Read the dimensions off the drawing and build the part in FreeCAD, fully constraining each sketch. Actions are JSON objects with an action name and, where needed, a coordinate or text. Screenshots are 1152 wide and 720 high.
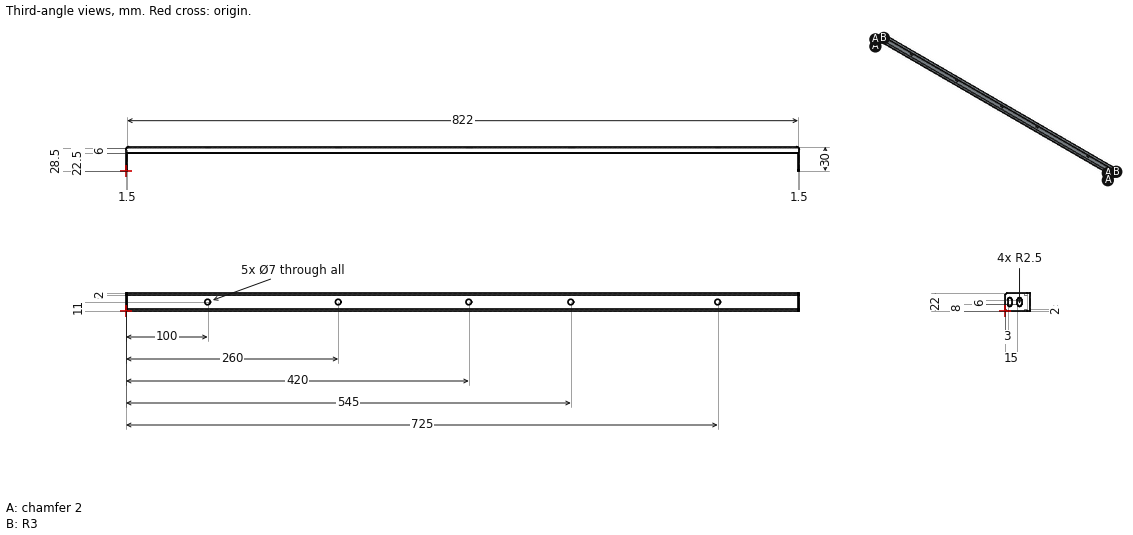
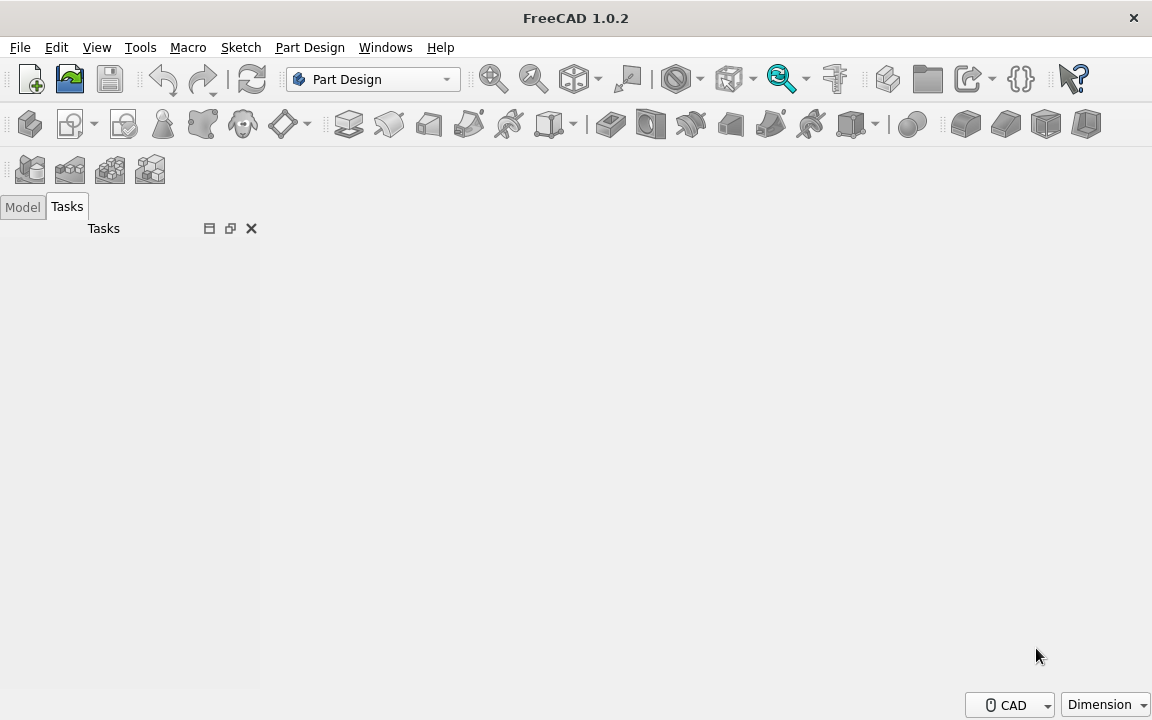
{"action": "left_click", "coordinate": [30, 80]}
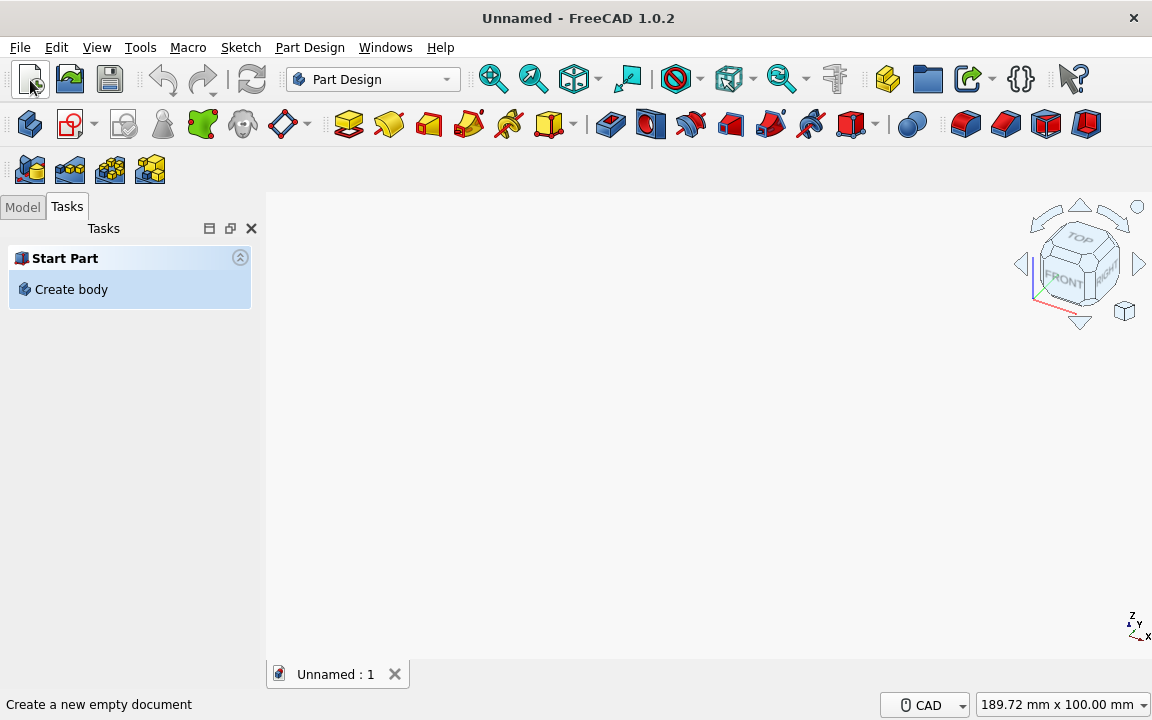
{"action": "left_click", "coordinate": [70, 124]}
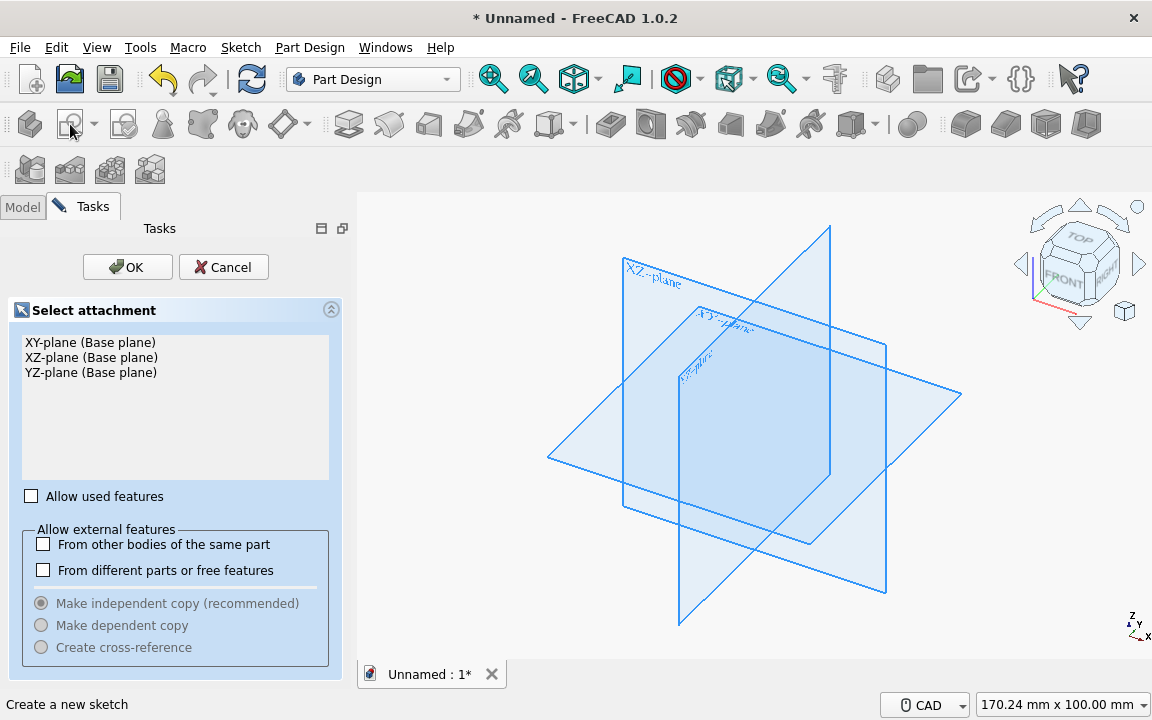
{"action": "left_click", "coordinate": [82, 342]}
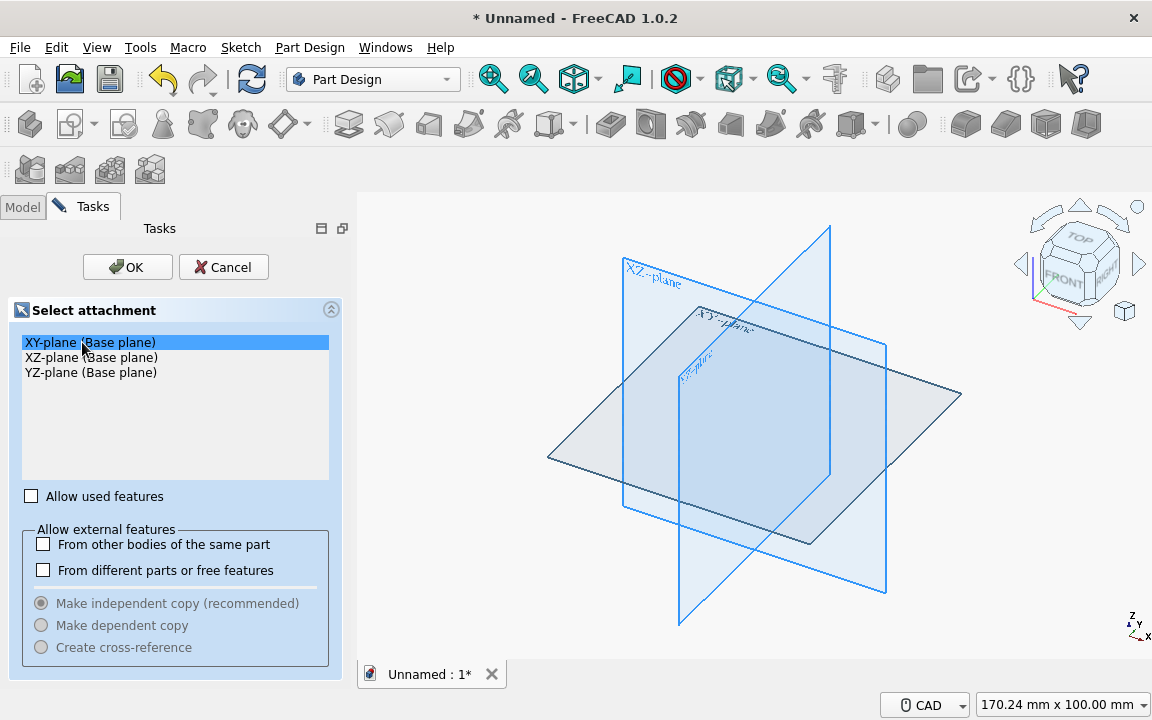
{"action": "left_click", "coordinate": [128, 267]}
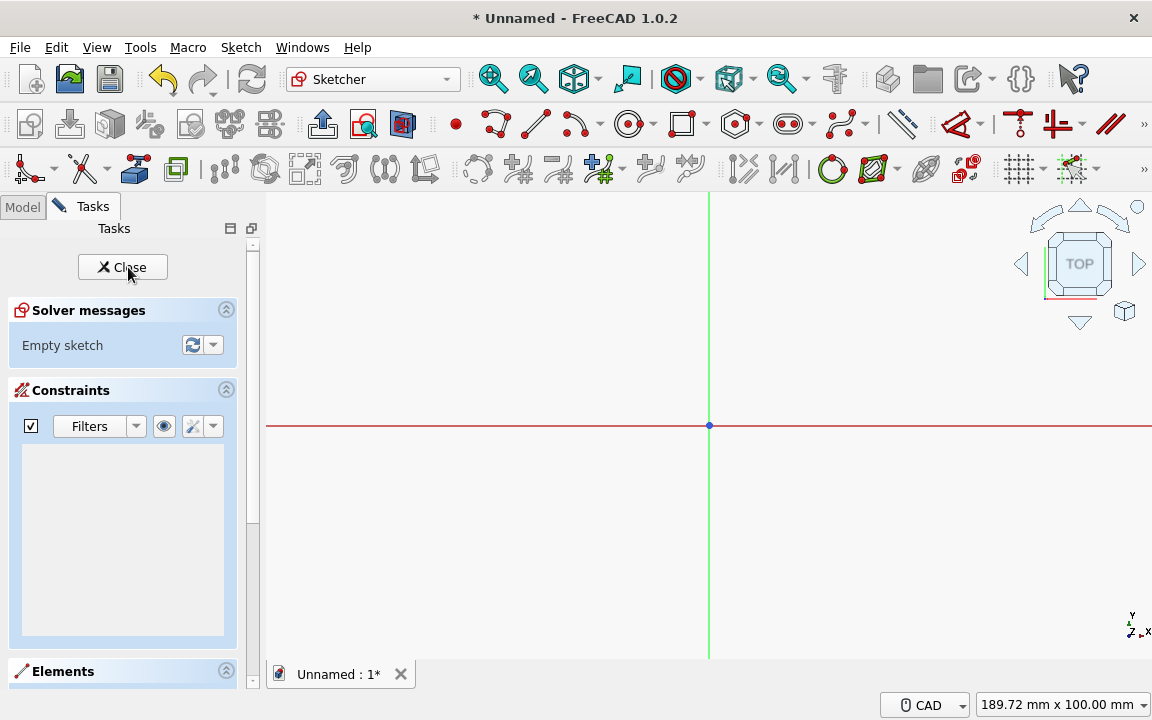
{"action": "scroll", "coordinate": [328, 436], "scroll_direction": "down", "scroll_amount": 10}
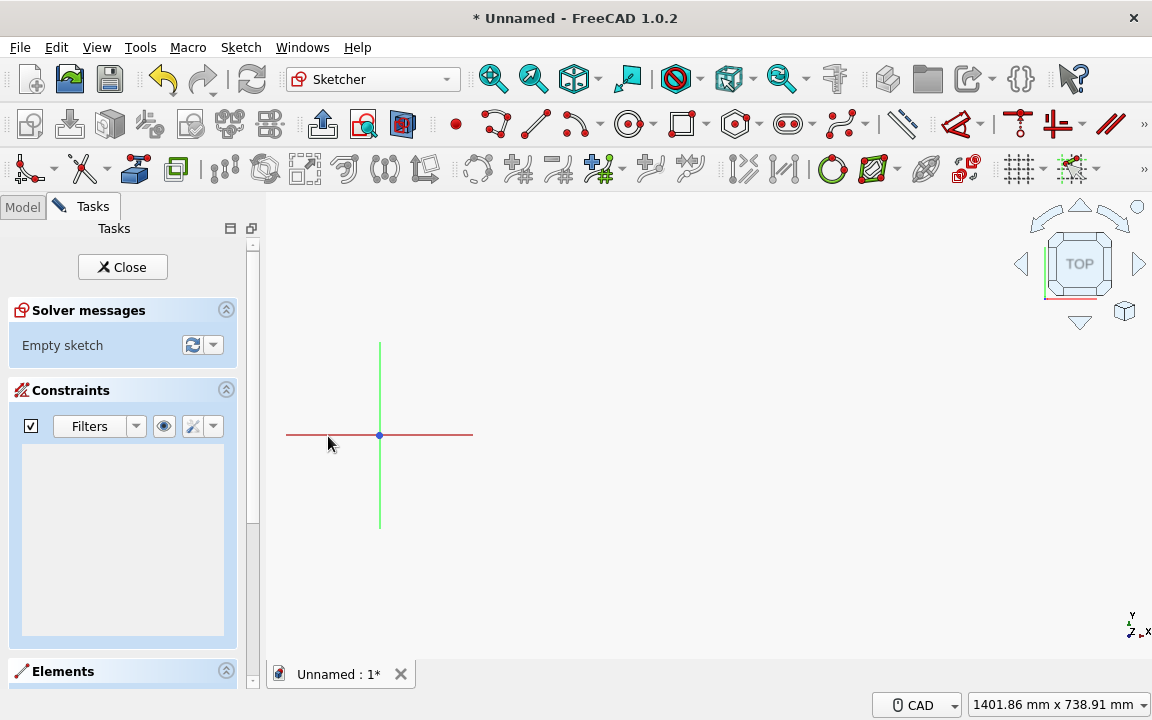
{"action": "left_click", "coordinate": [496, 124]}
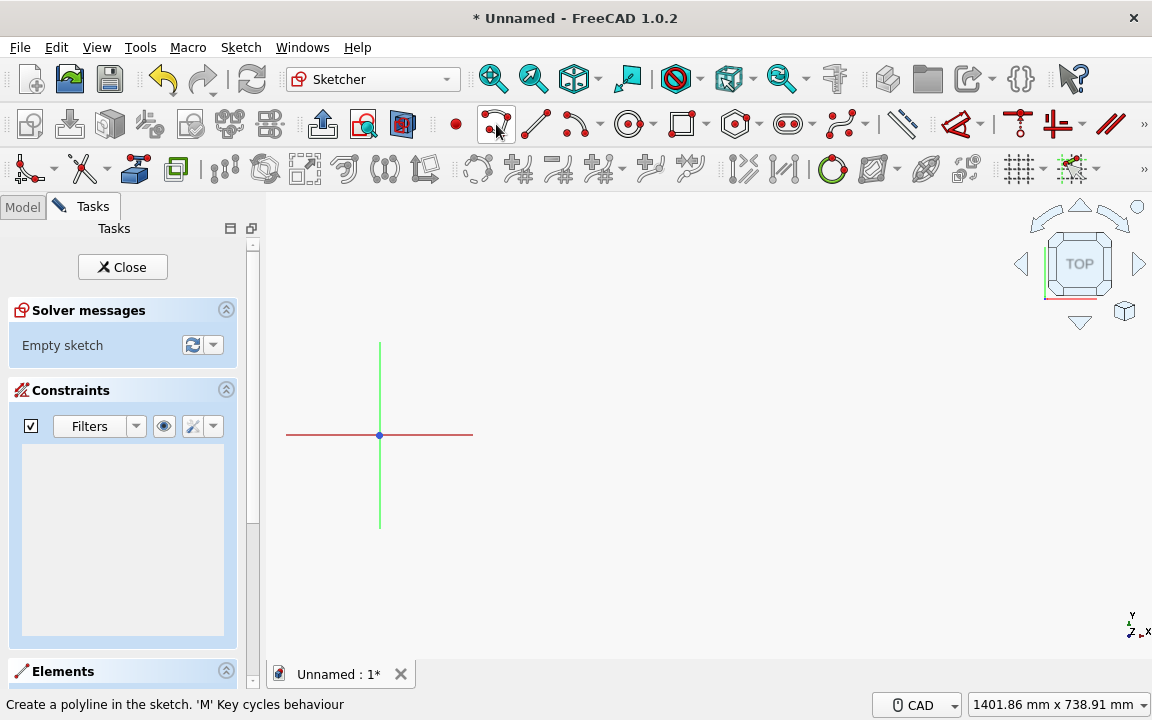
{"action": "left_click", "coordinate": [380, 435]}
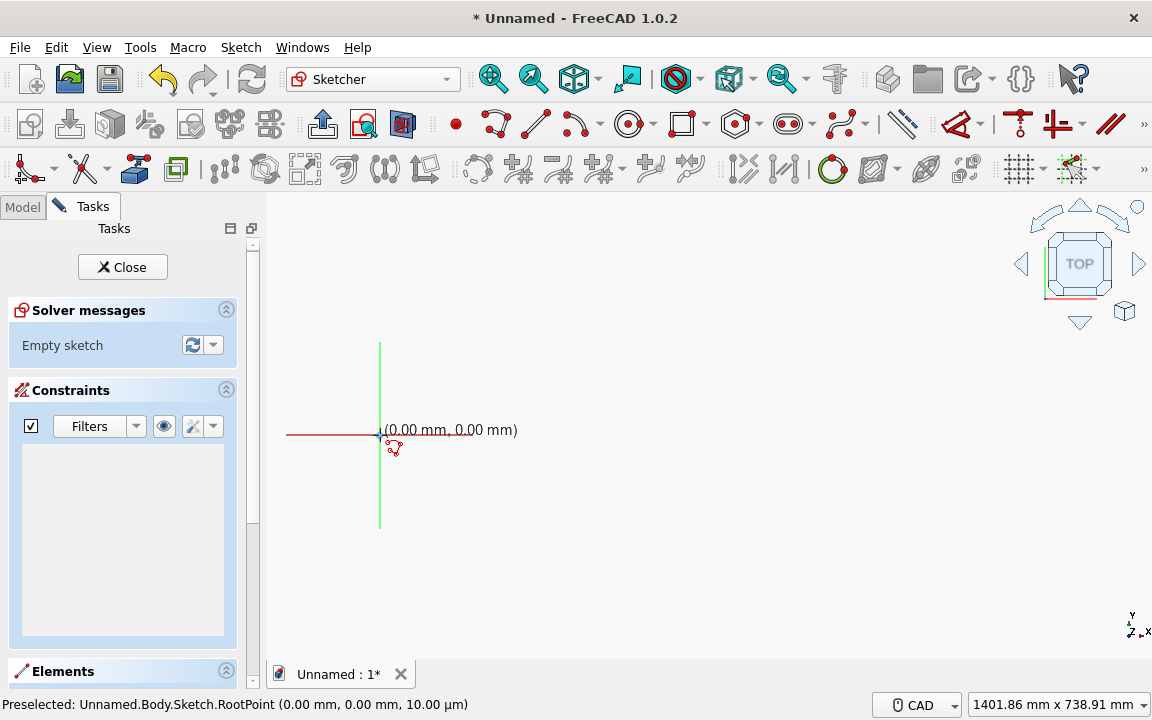
{"action": "scroll", "coordinate": [381, 435], "scroll_direction": "up", "scroll_amount": 15}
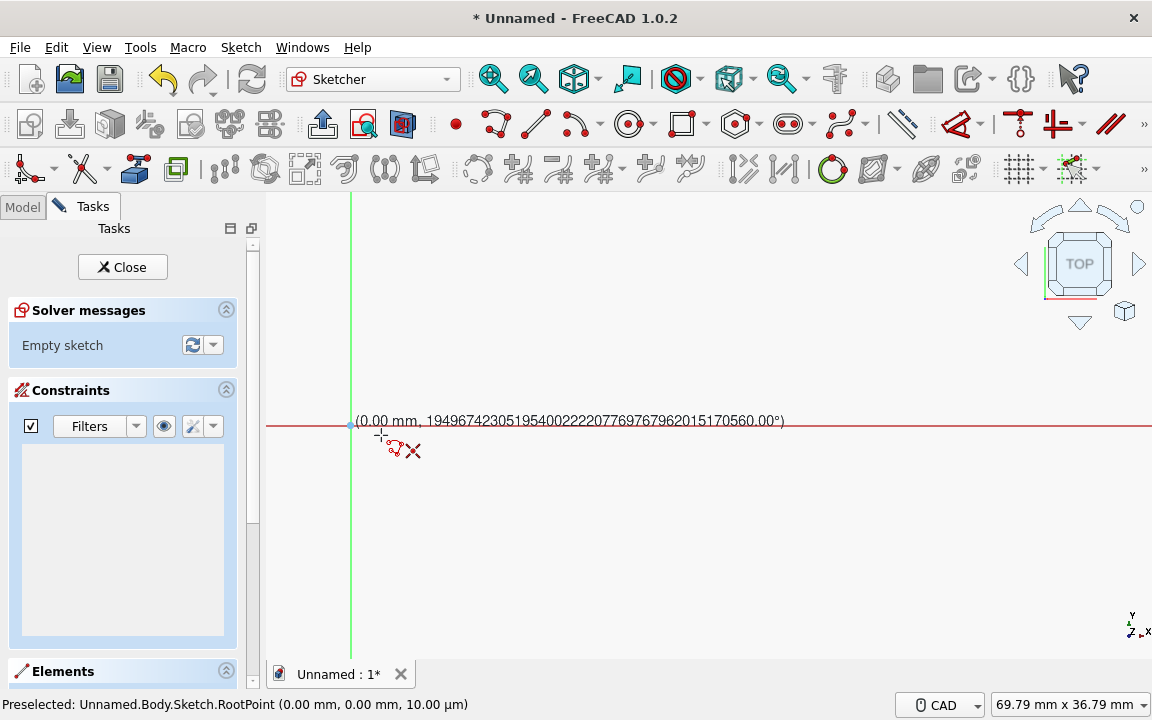
{"action": "left_click", "coordinate": [370, 417]}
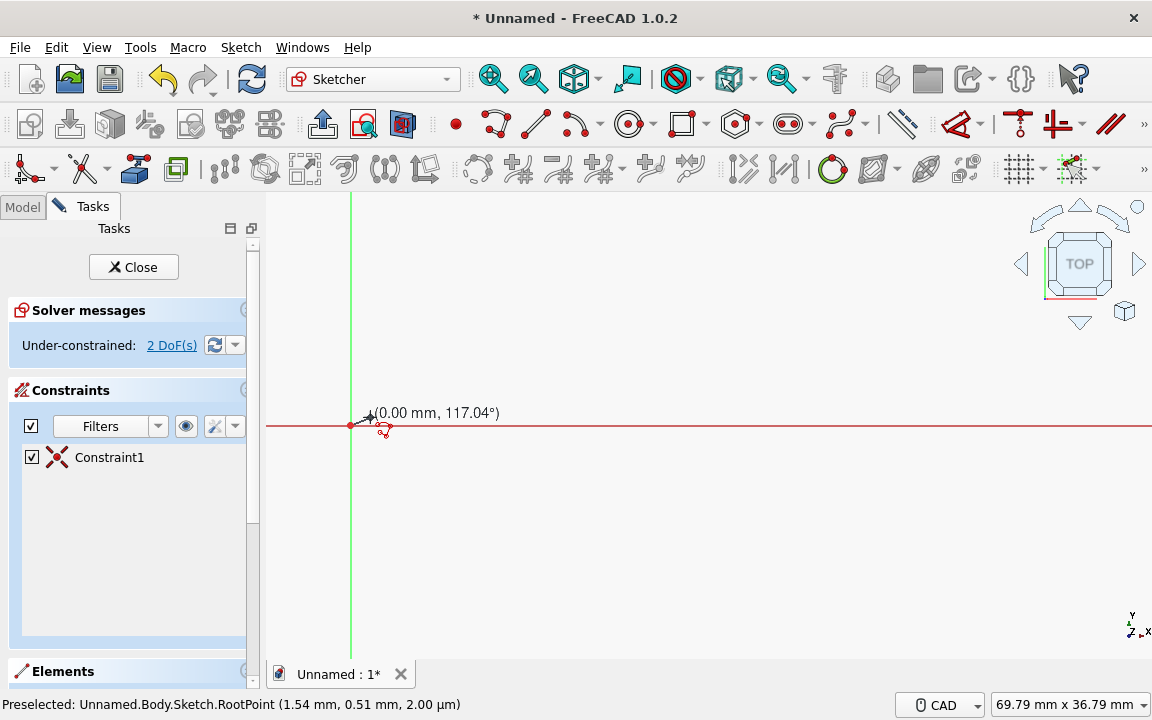
{"action": "scroll", "coordinate": [381, 435], "scroll_direction": "down", "scroll_amount": 15}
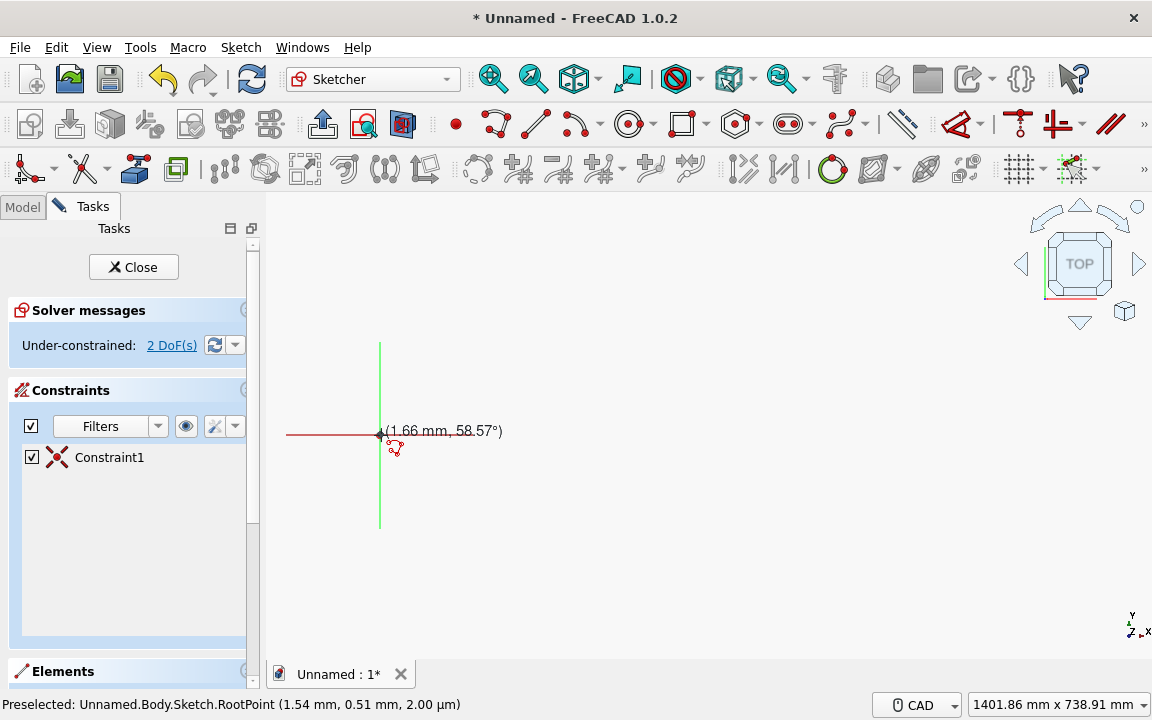
{"action": "scroll", "coordinate": [381, 417], "scroll_direction": "up", "scroll_amount": 15}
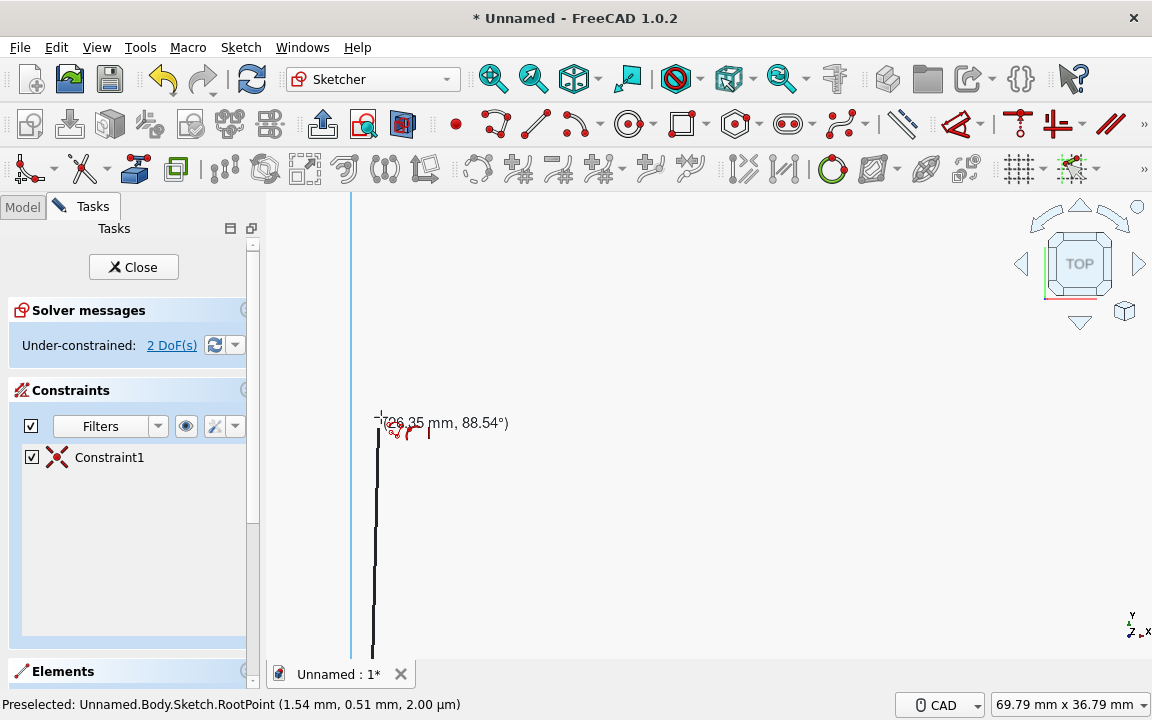
{"action": "left_click", "coordinate": [370, 408]}